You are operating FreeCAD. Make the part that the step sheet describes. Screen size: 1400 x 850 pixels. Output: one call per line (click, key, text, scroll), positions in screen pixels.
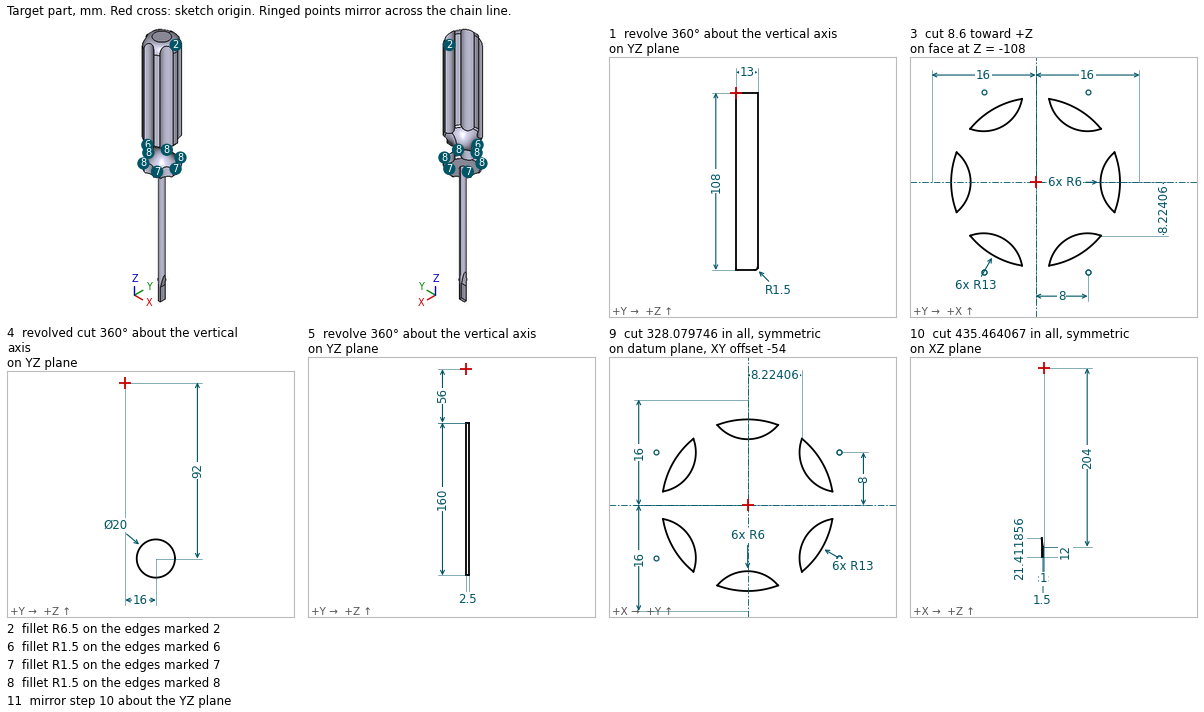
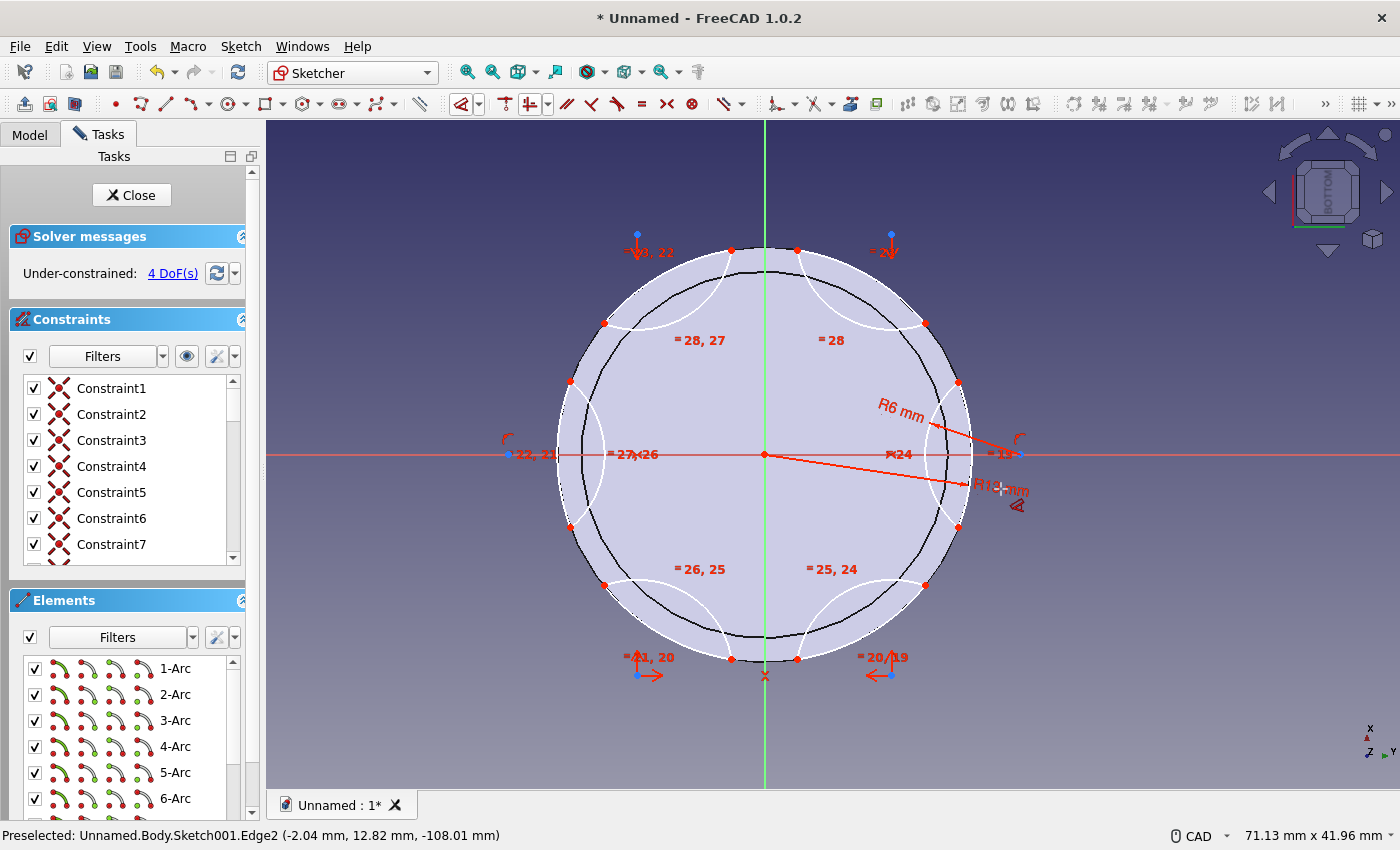
click(892, 676)
click(828, 710)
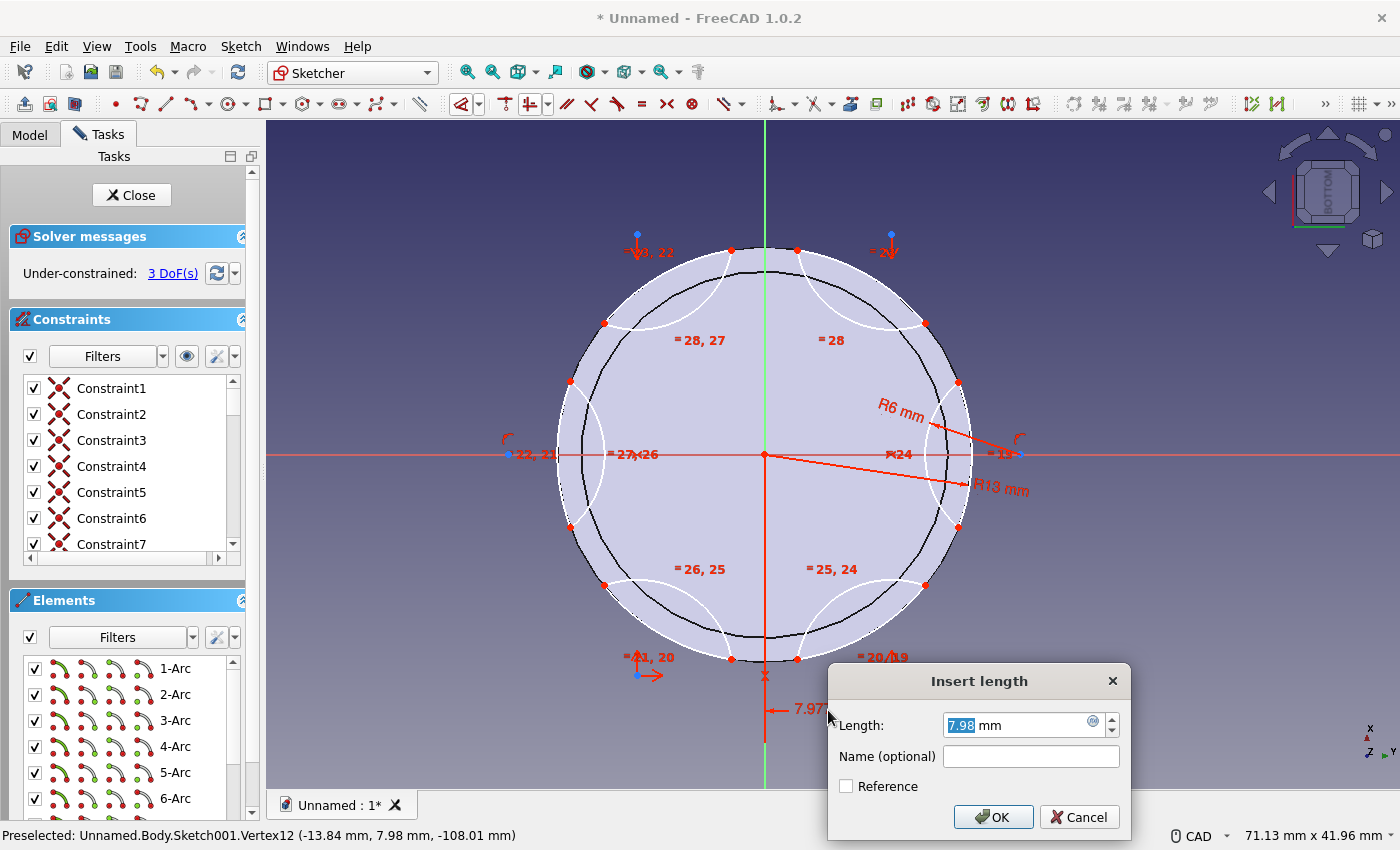
text(8)
key(Return)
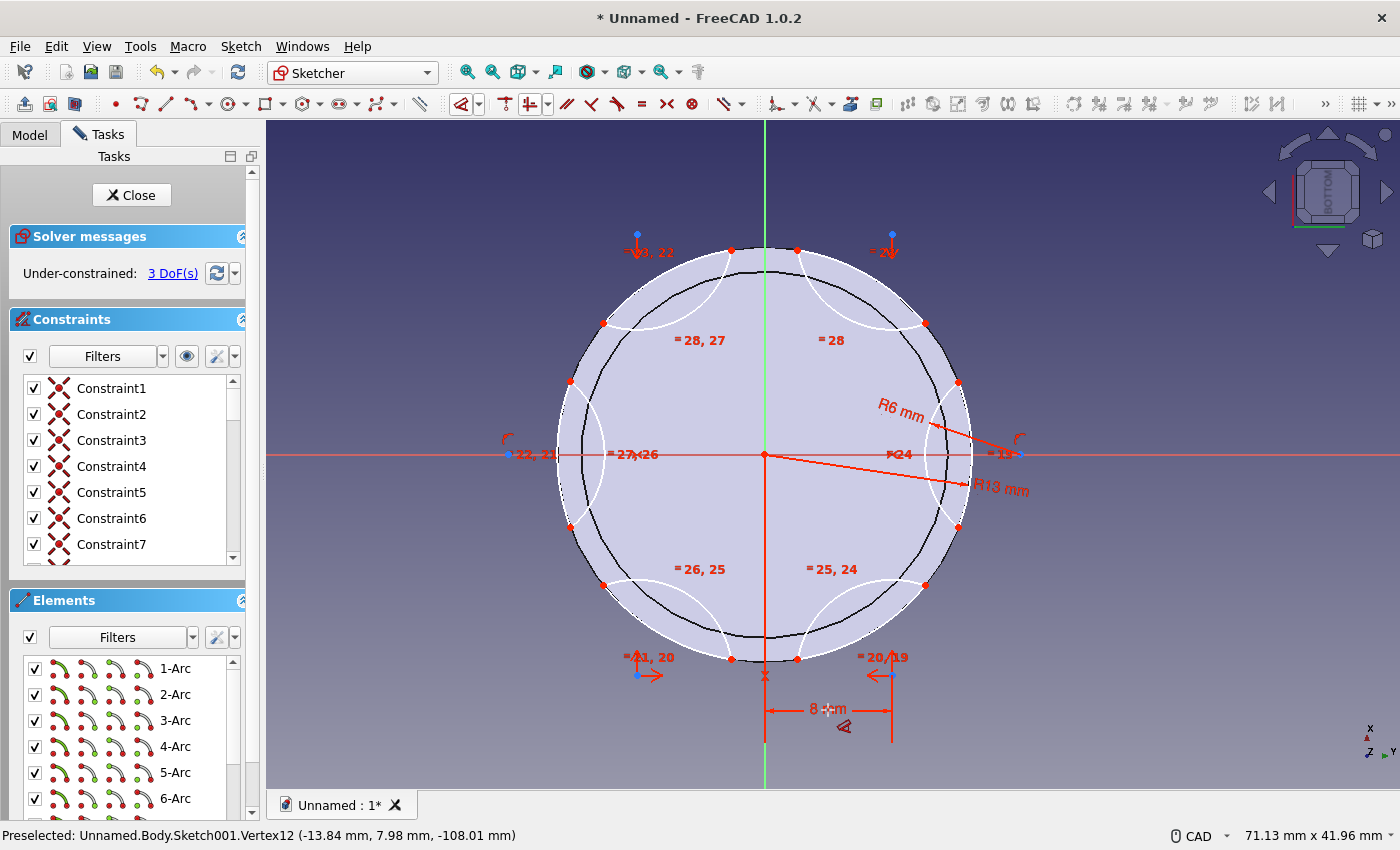
click(1021, 455)
click(893, 489)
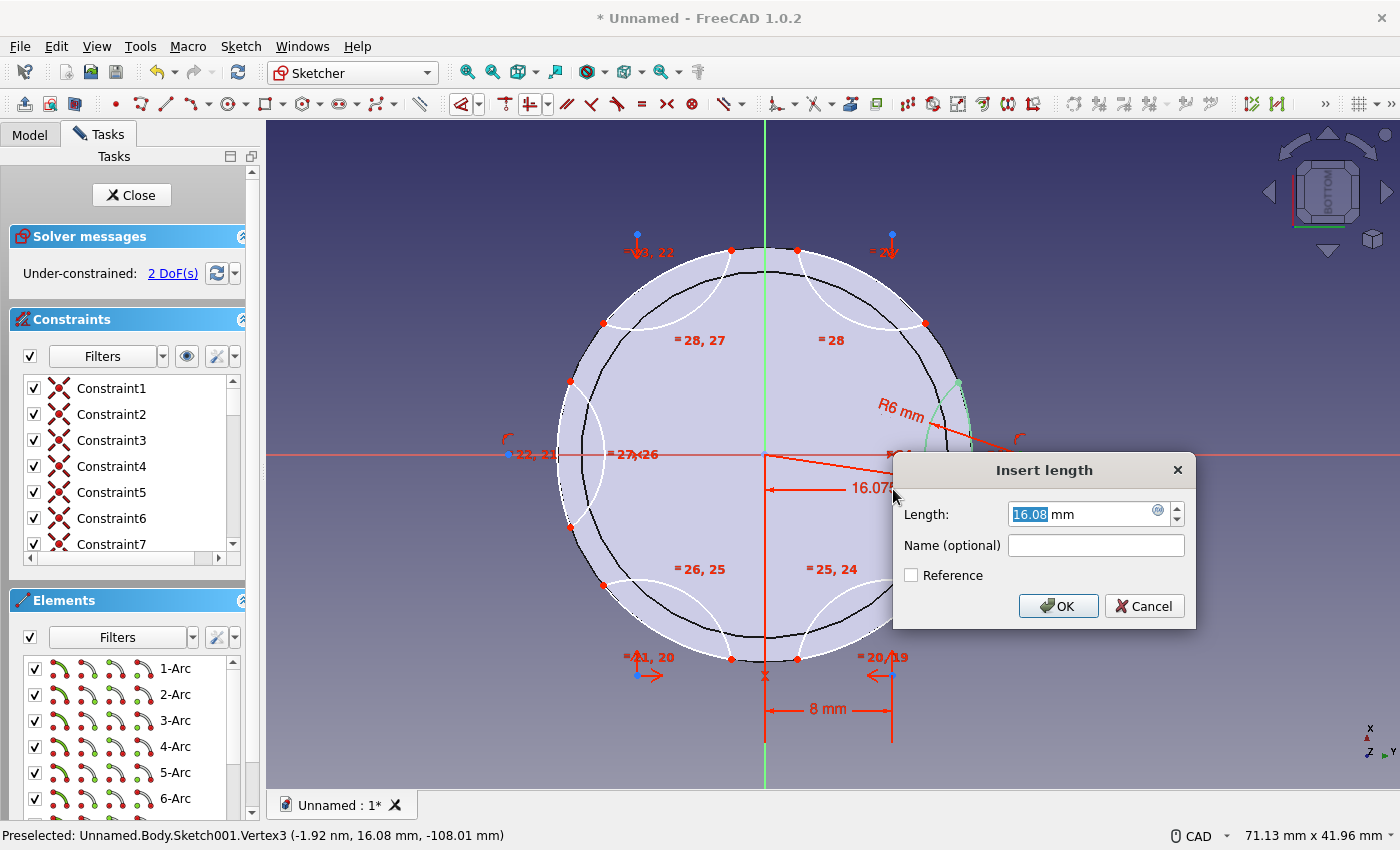
text(16)
key(Return)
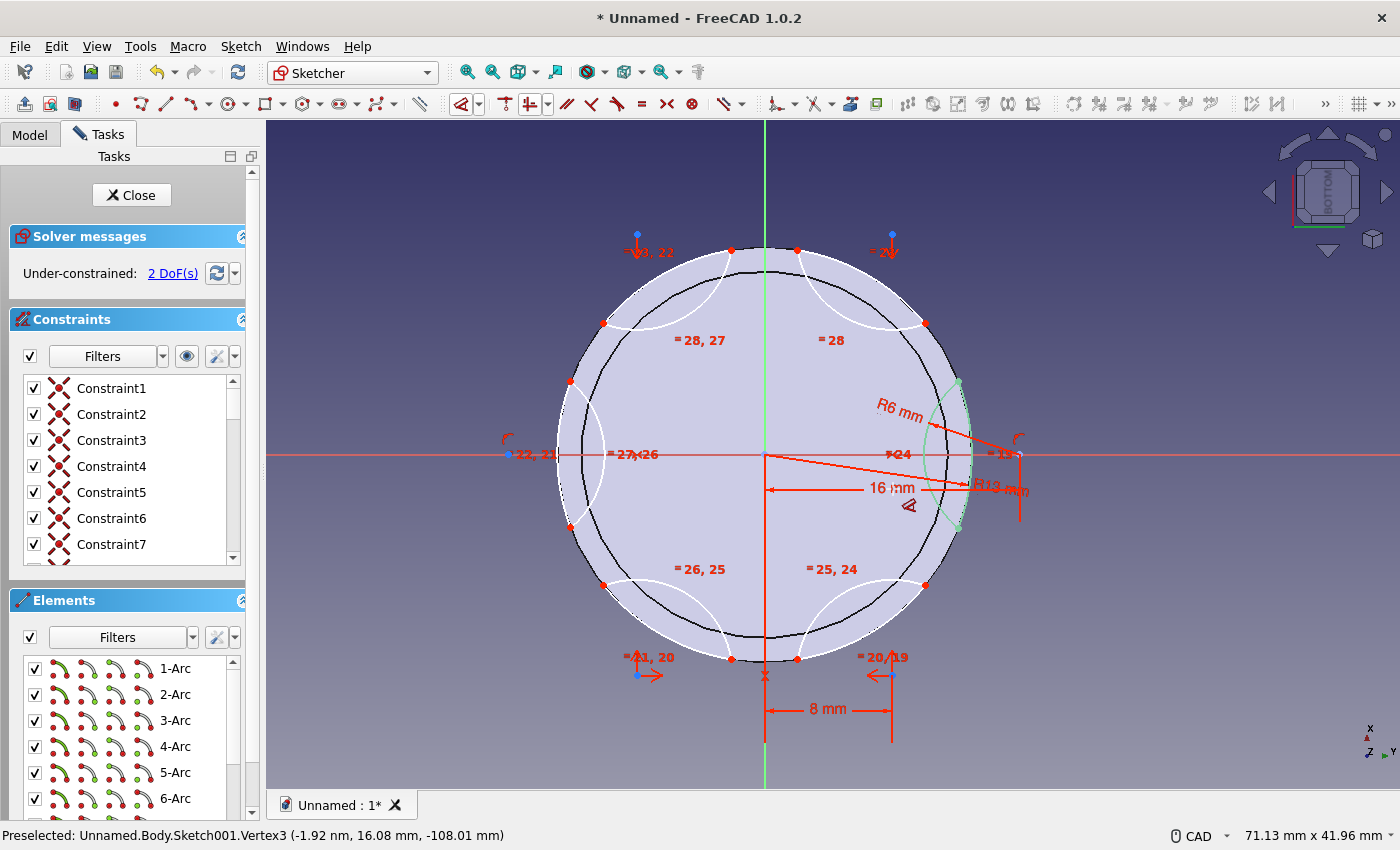
click(509, 455)
click(637, 489)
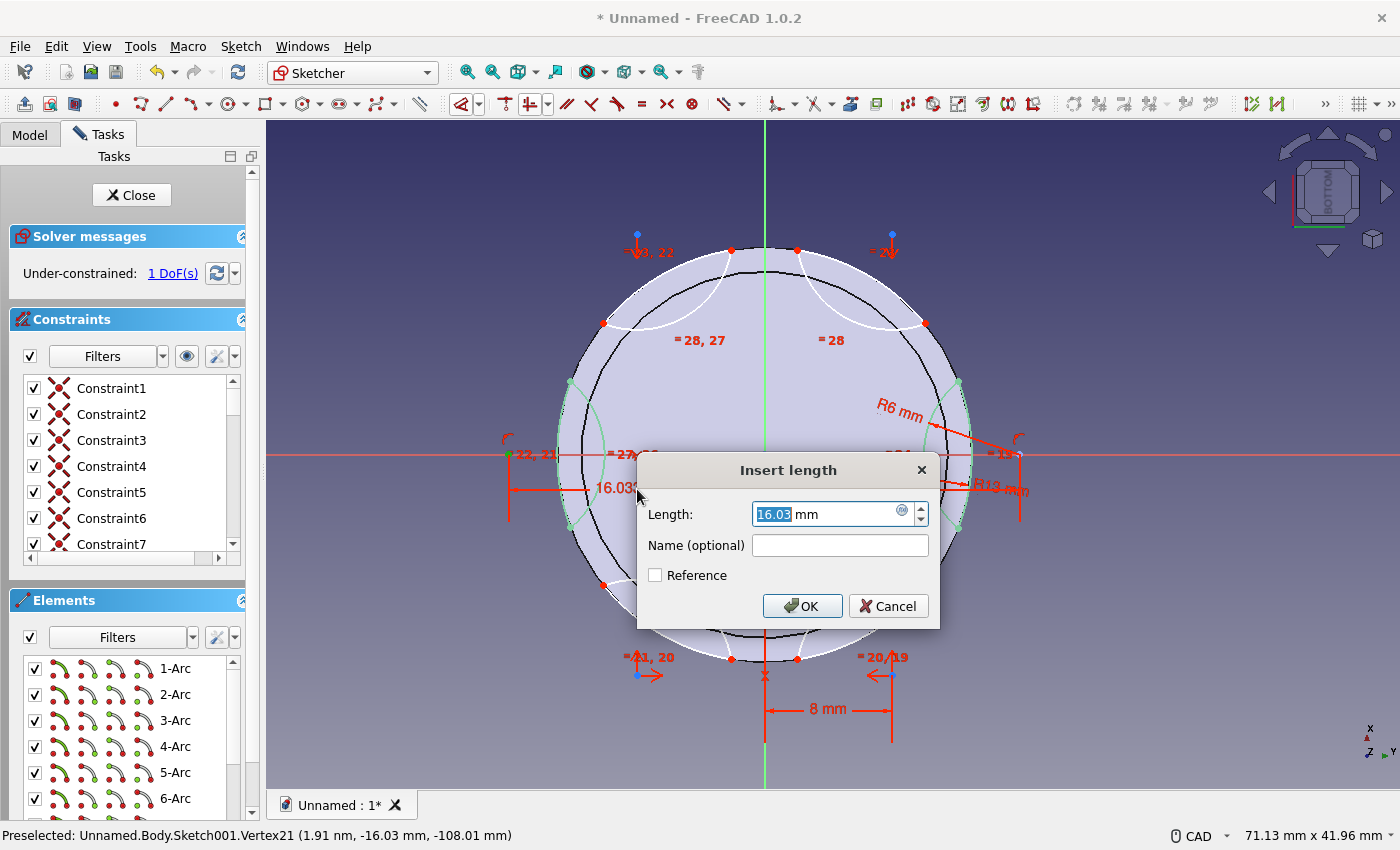
text(16)
key(Return)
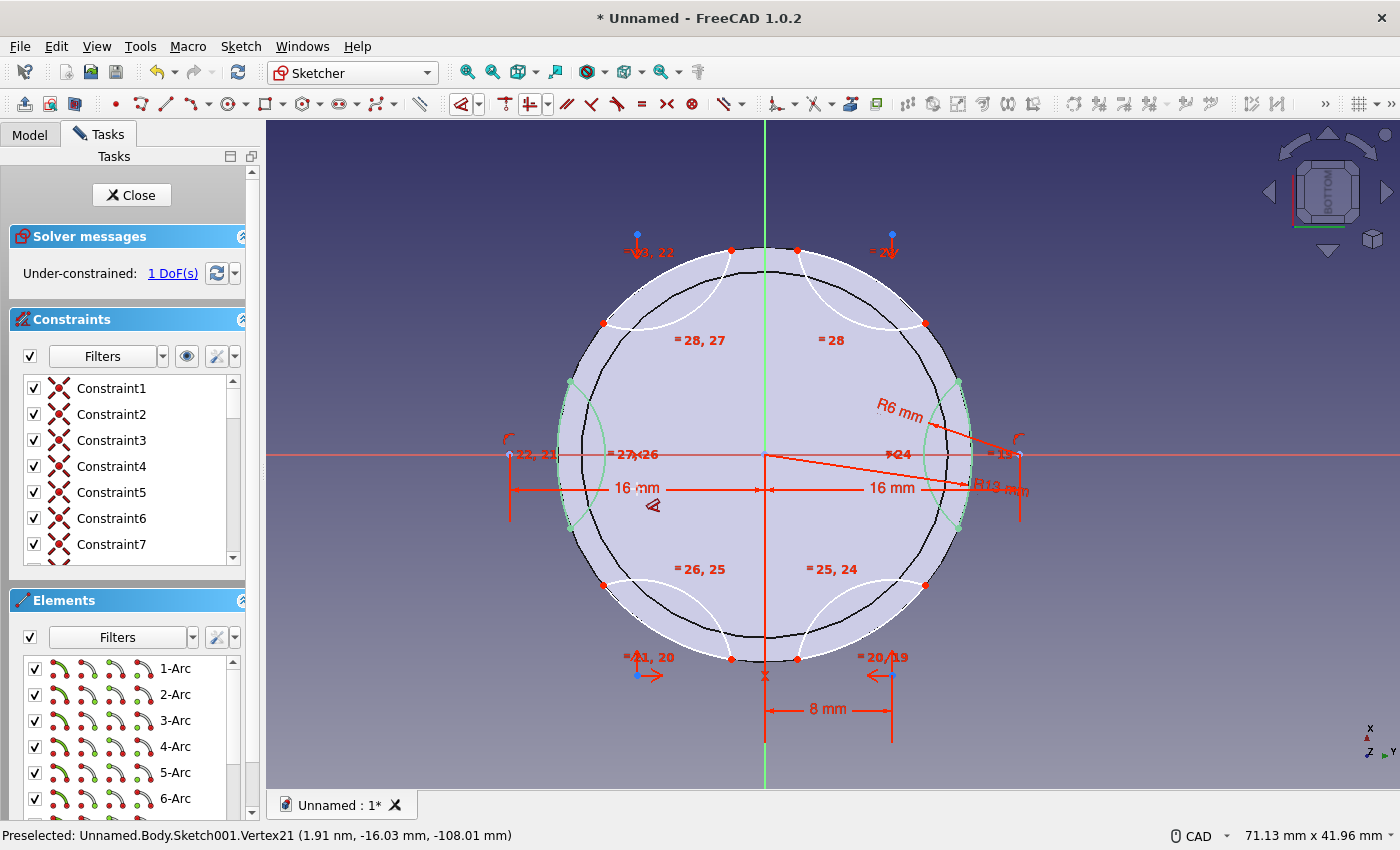
click(925, 586)
click(959, 550)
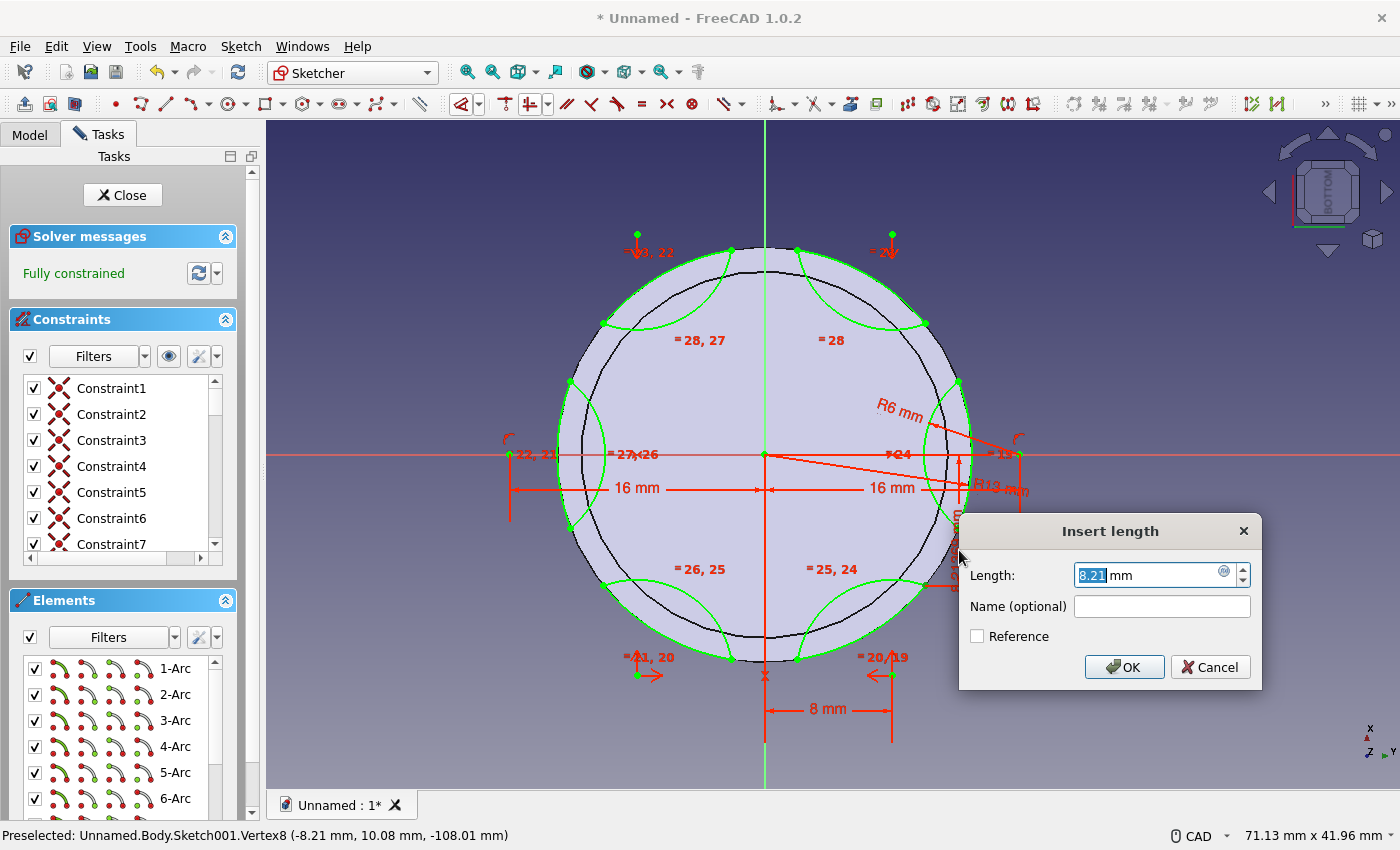
text(8.22406)
key(Return)
key(Escape)